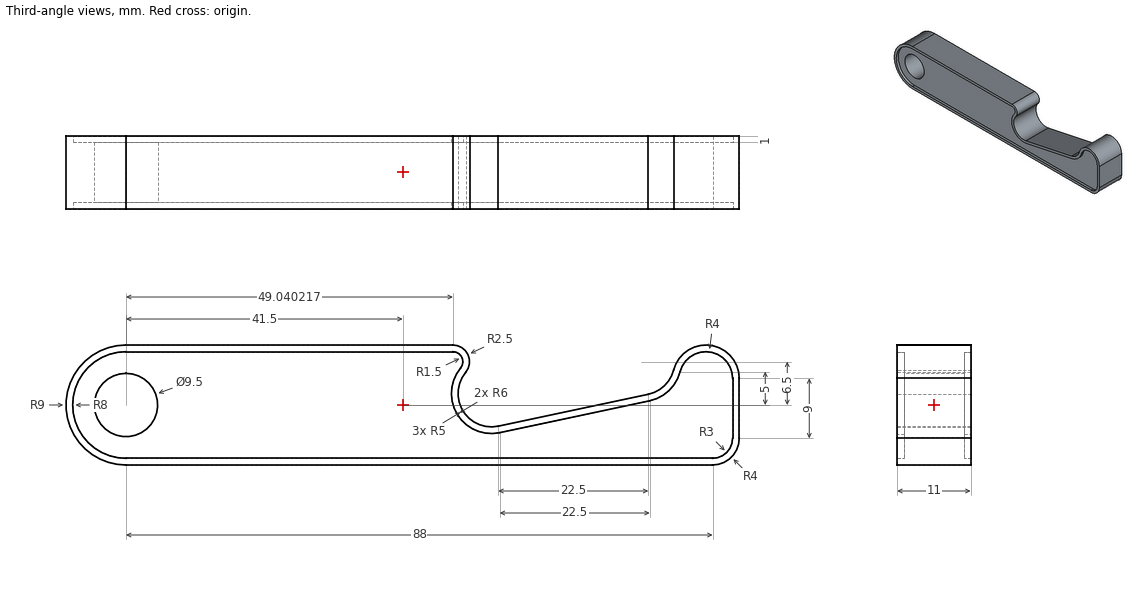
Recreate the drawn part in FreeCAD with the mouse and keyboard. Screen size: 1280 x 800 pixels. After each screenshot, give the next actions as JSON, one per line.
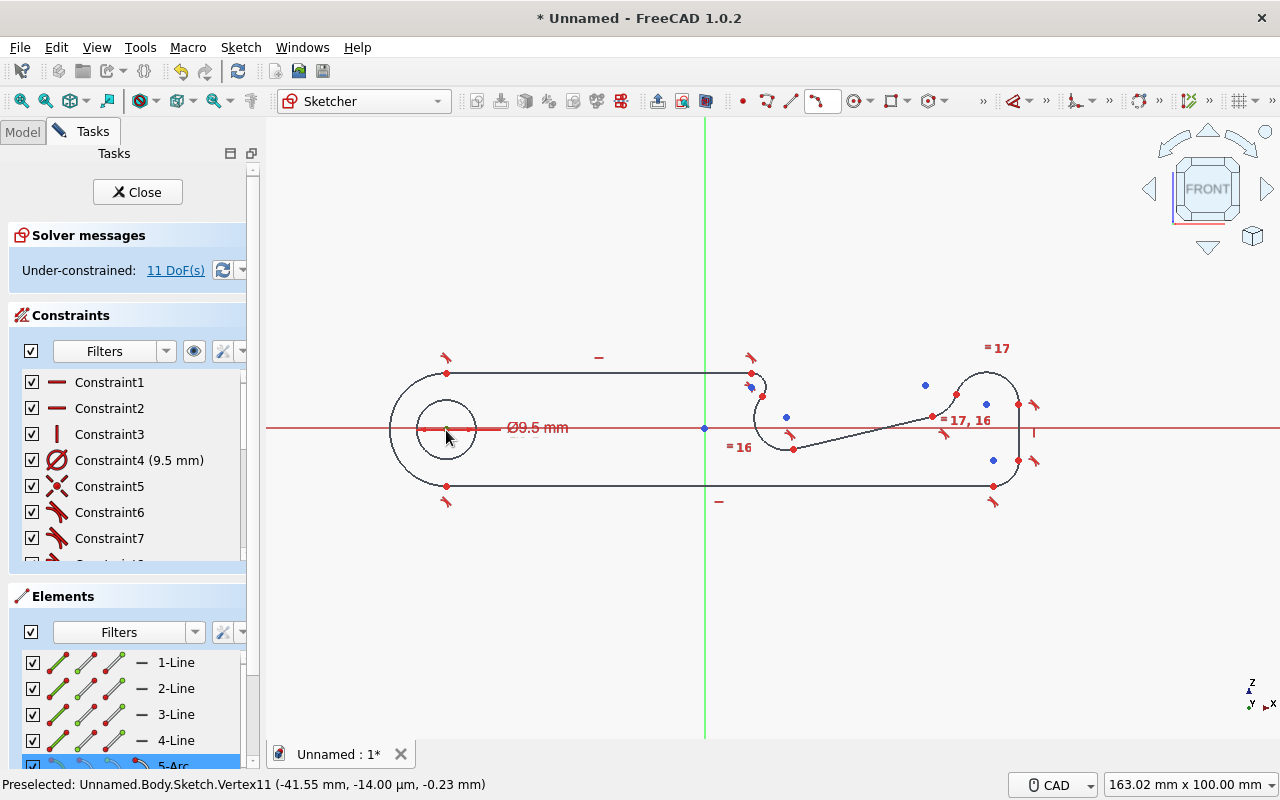
{"action": "left_click", "coordinate": [353, 428]}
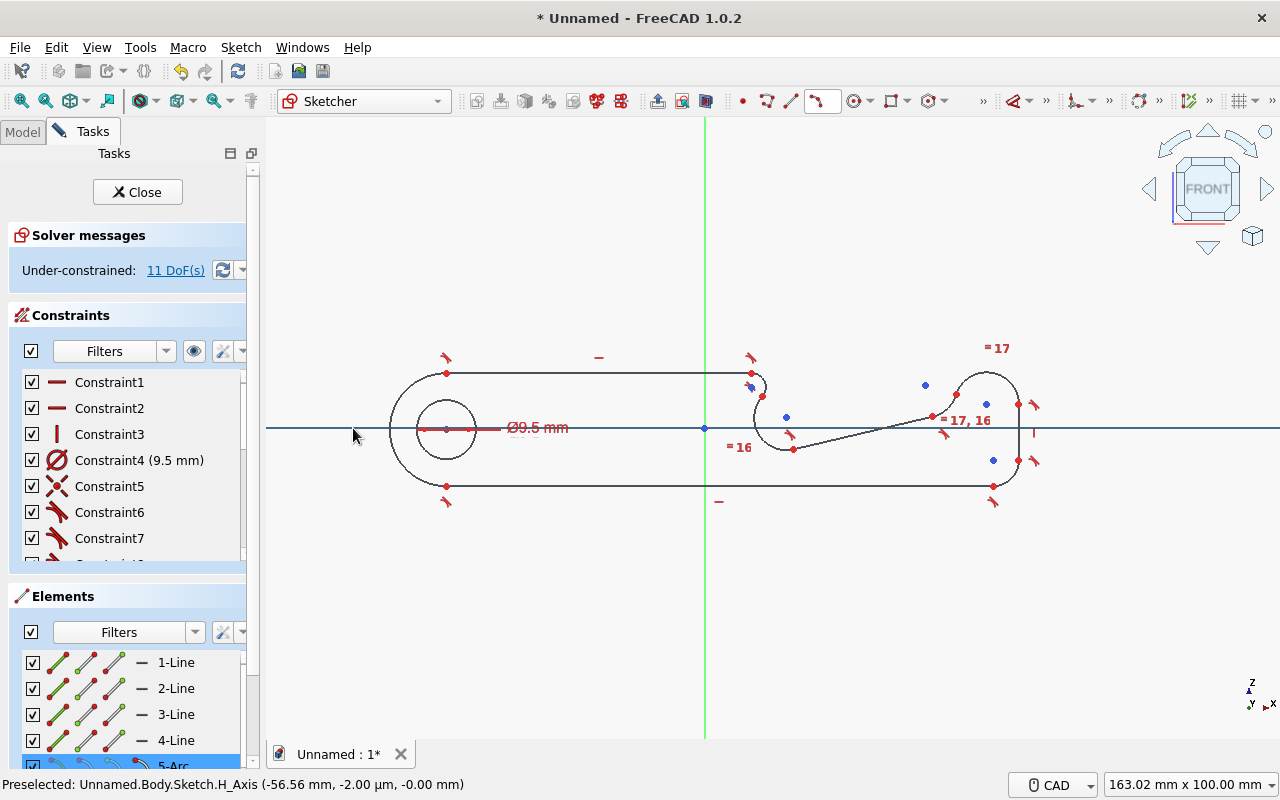
{"action": "key", "text": "c"}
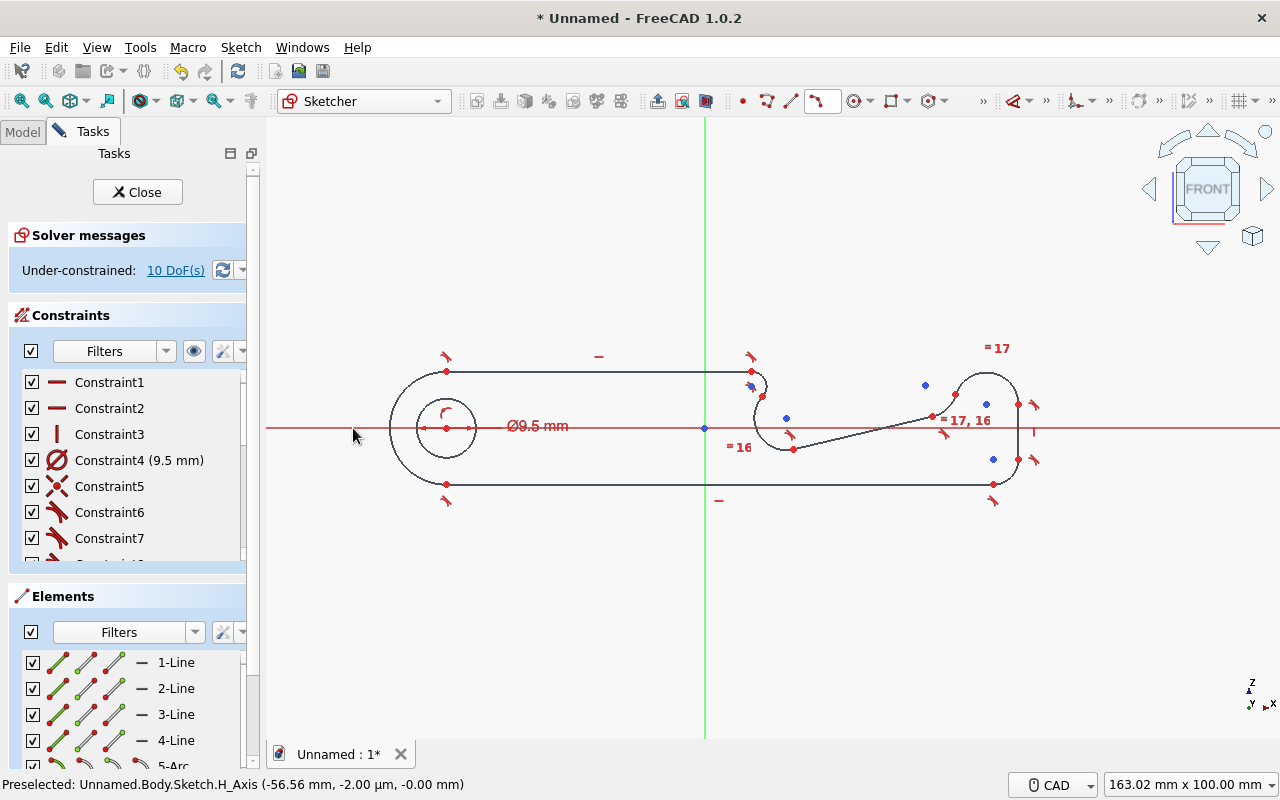
{"action": "left_click", "coordinate": [1014, 102]}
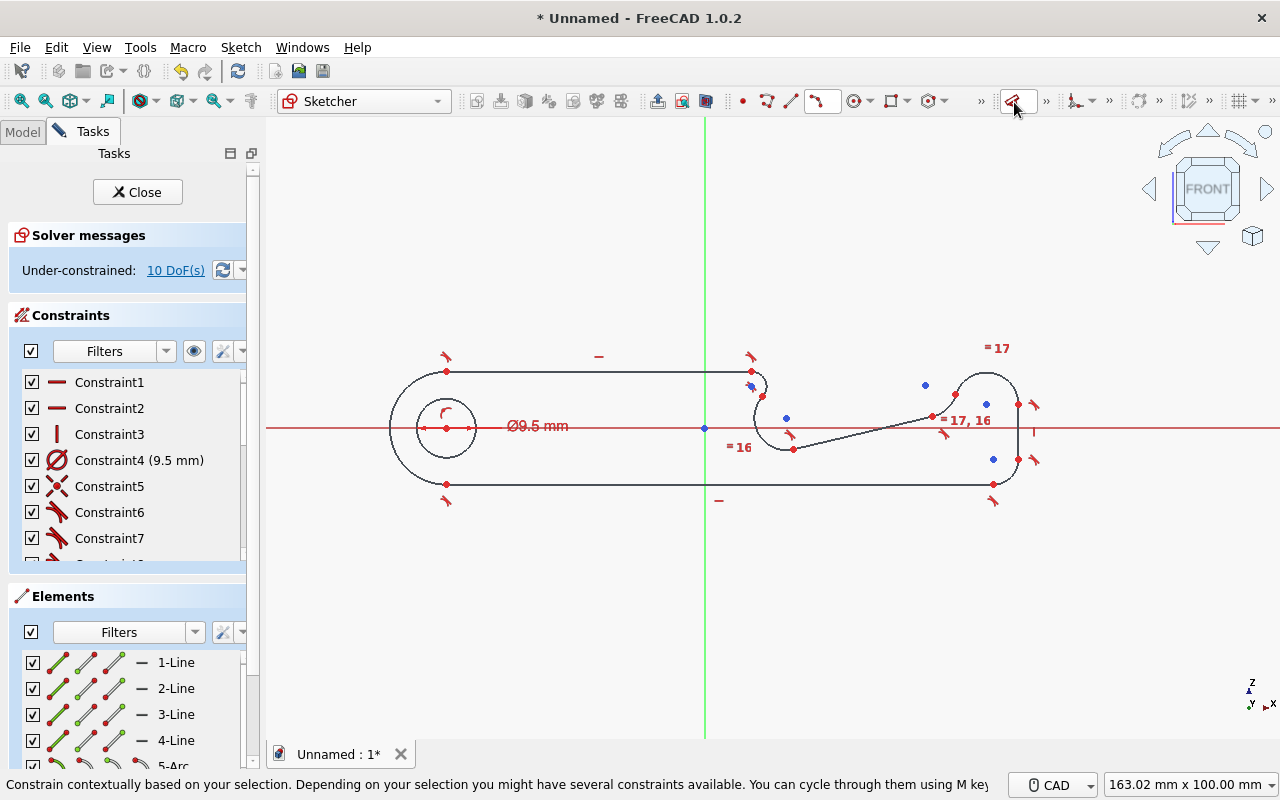
{"action": "left_click", "coordinate": [401, 395]}
{"action": "left_click", "coordinate": [375, 376]}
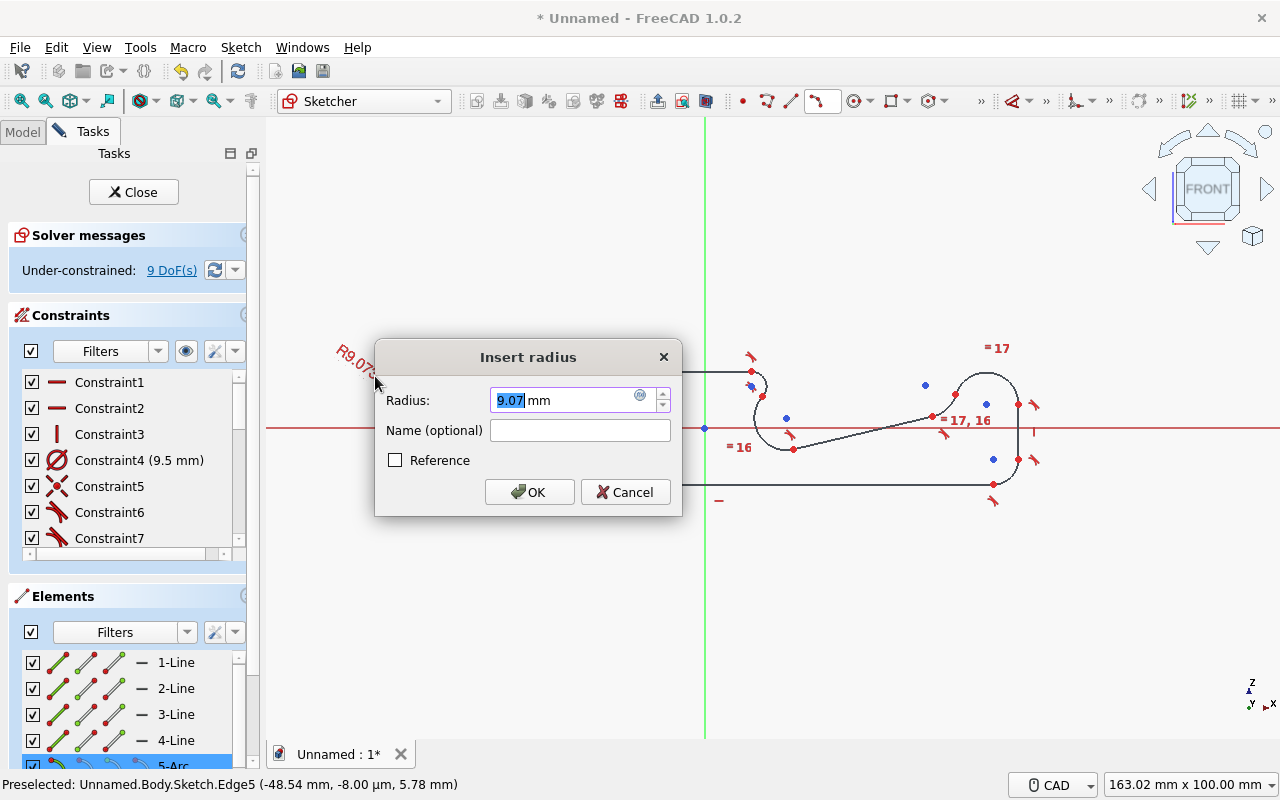
{"action": "type", "text": "9"}
{"action": "key", "text": "Return"}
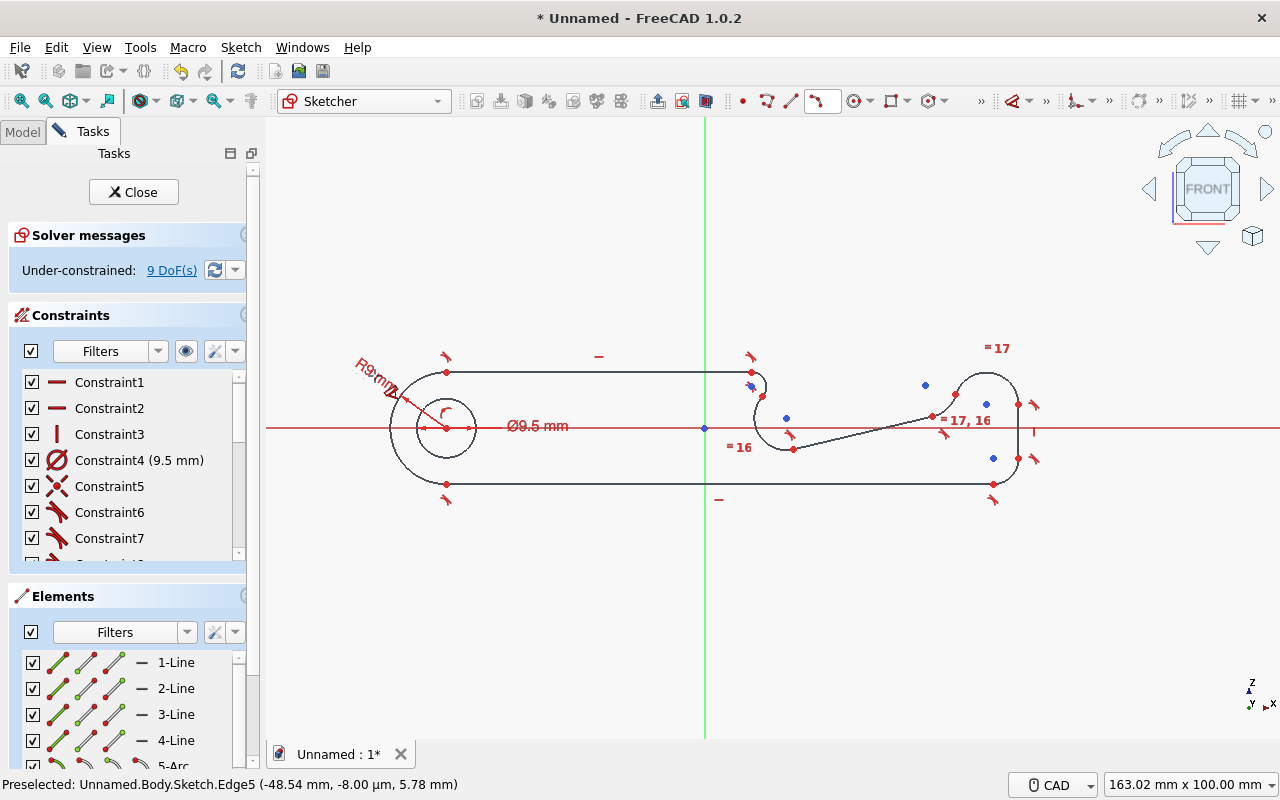
{"action": "scroll", "coordinate": [766, 387], "scroll_direction": "up", "scroll_amount": 5}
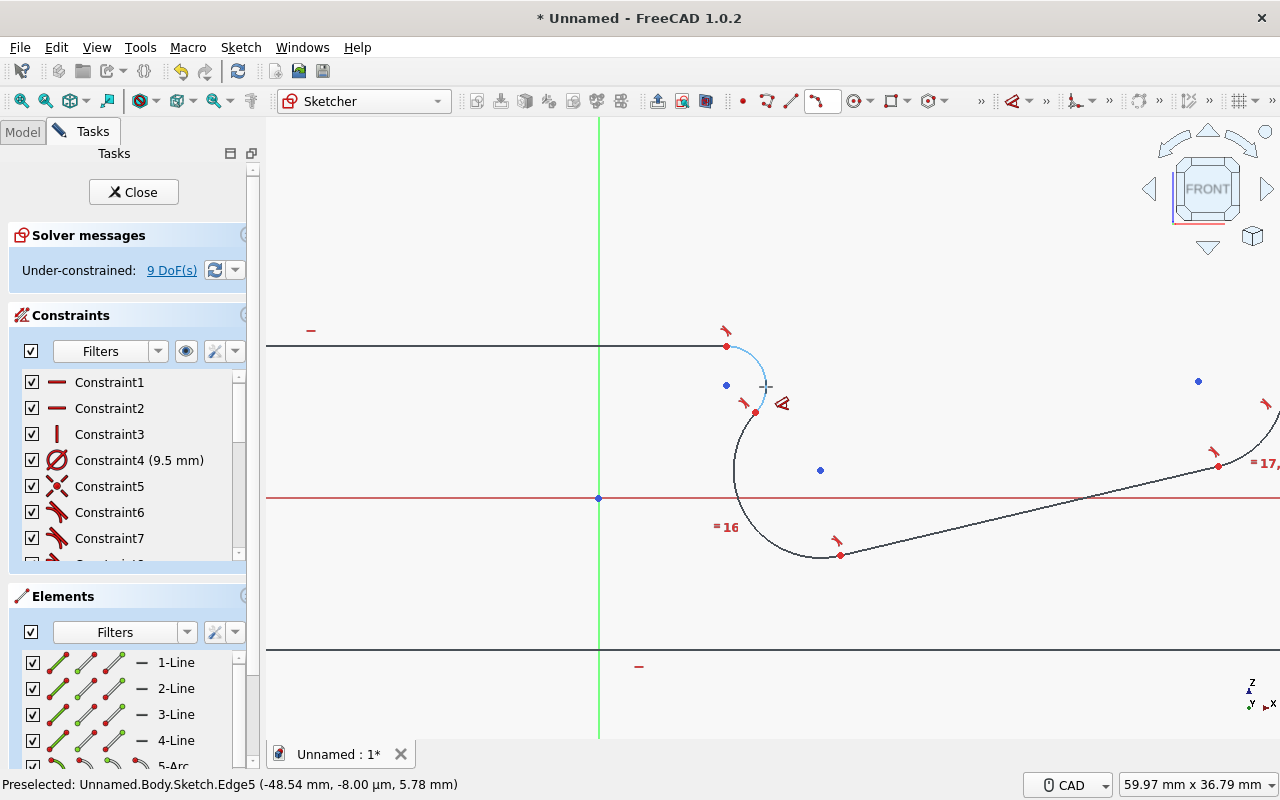
{"action": "left_click", "coordinate": [766, 388]}
{"action": "left_click", "coordinate": [798, 390]}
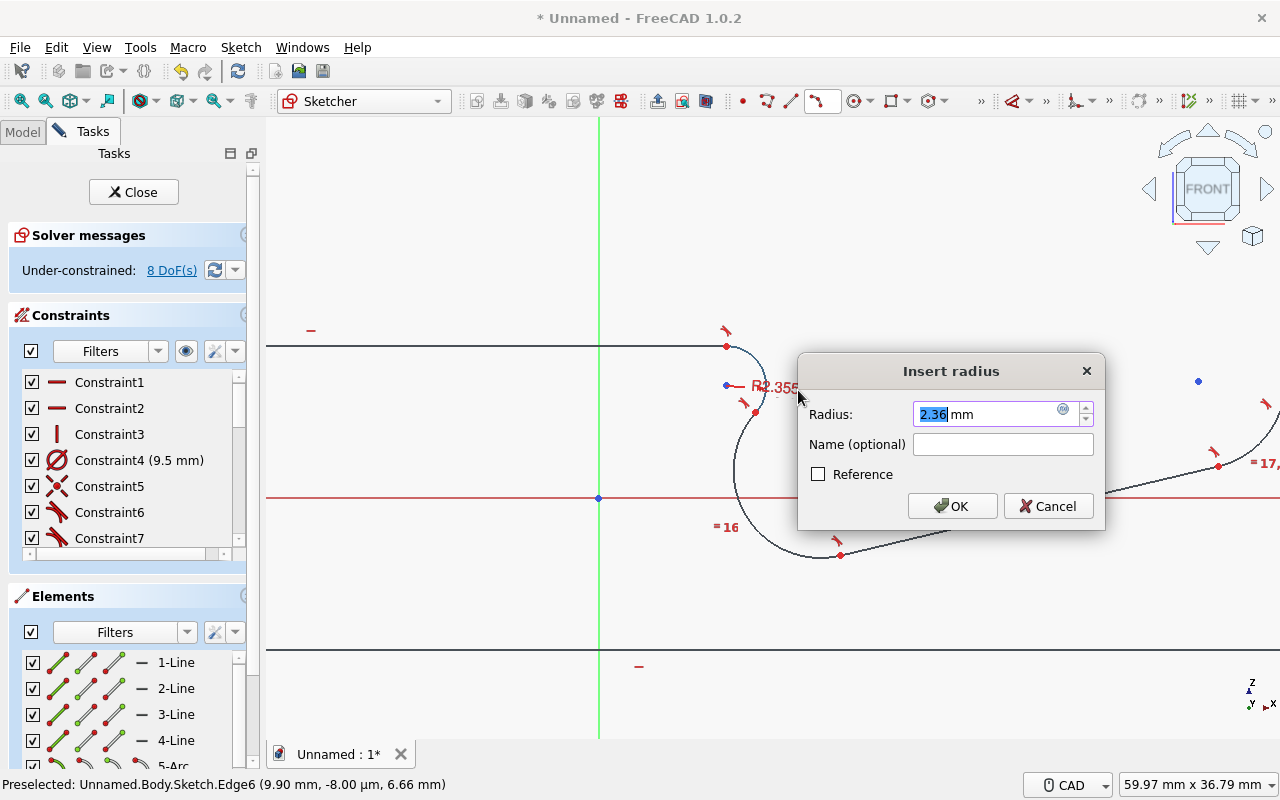
{"action": "type", "text": "2.5"}
{"action": "key", "text": "Return"}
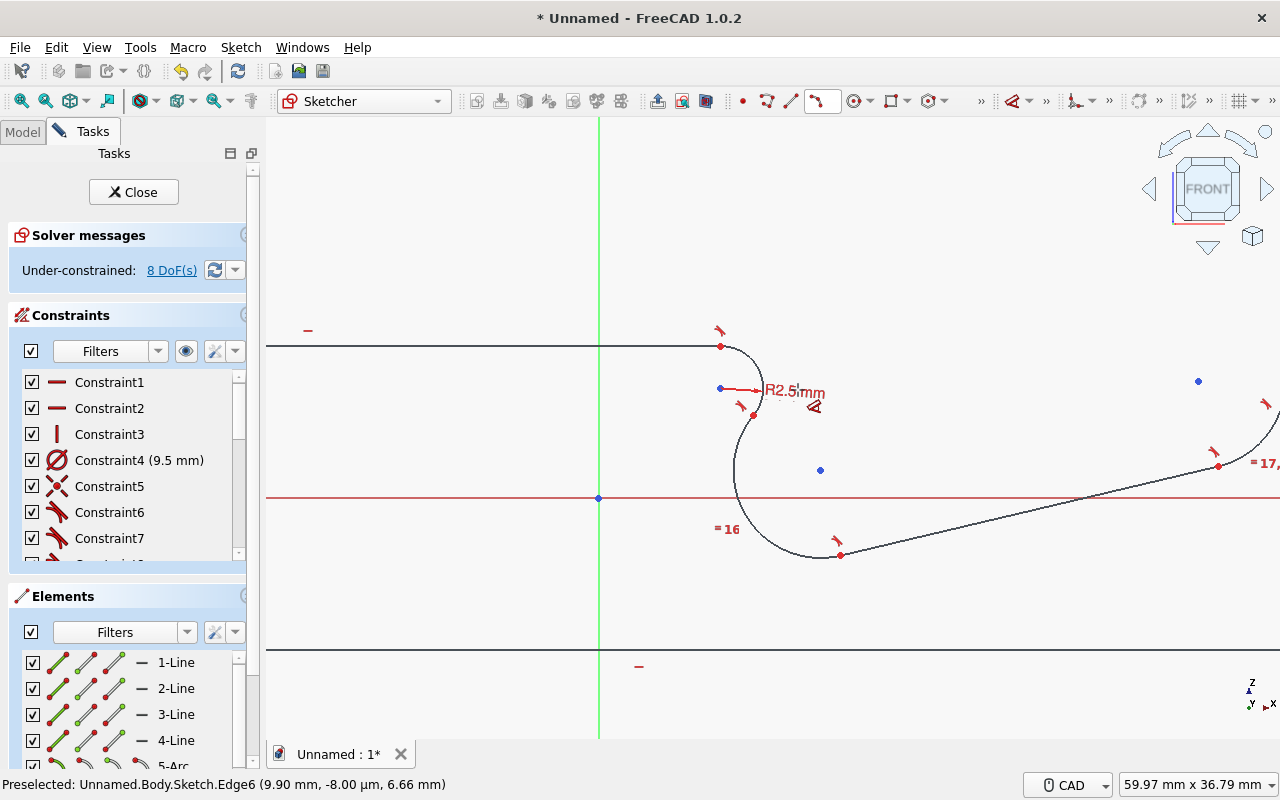
{"action": "left_click", "coordinate": [734, 476]}
{"action": "left_click", "coordinate": [702, 478]}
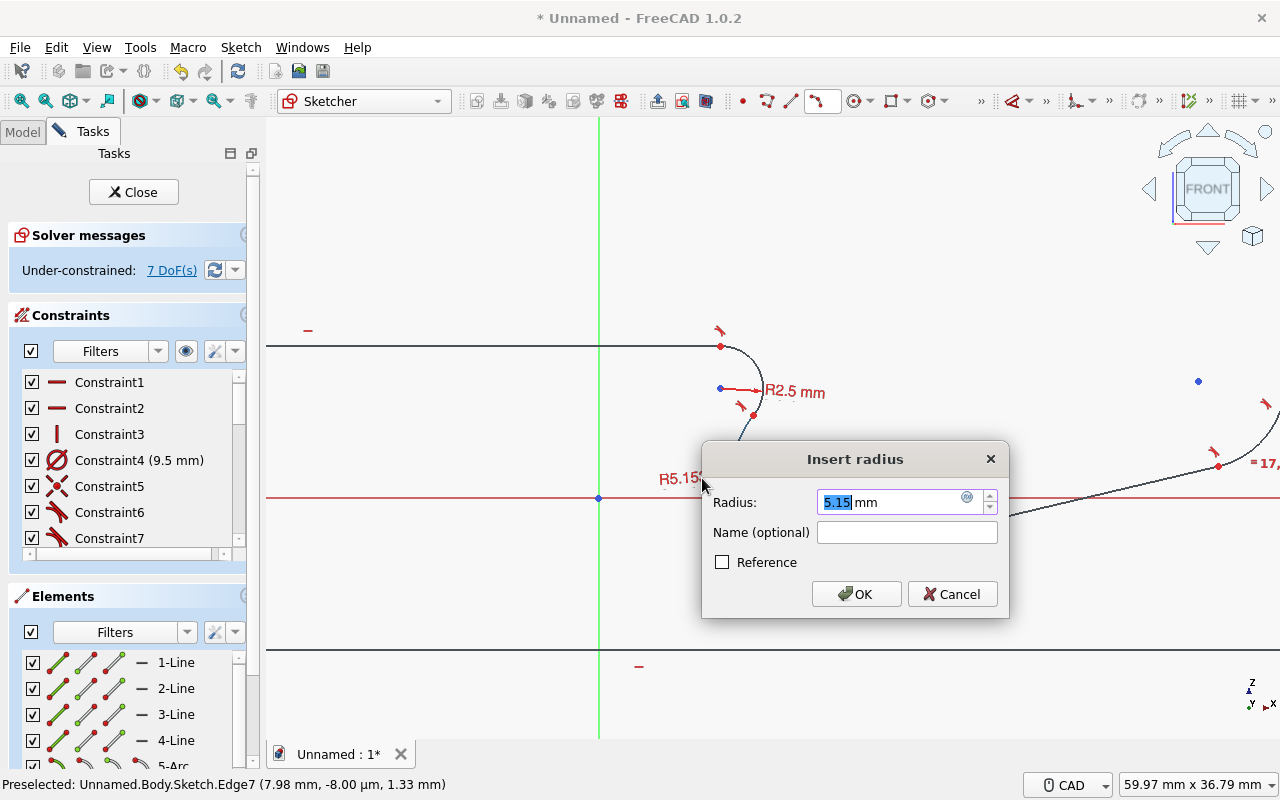
{"action": "type", "text": "5"}
{"action": "key", "text": "Return"}